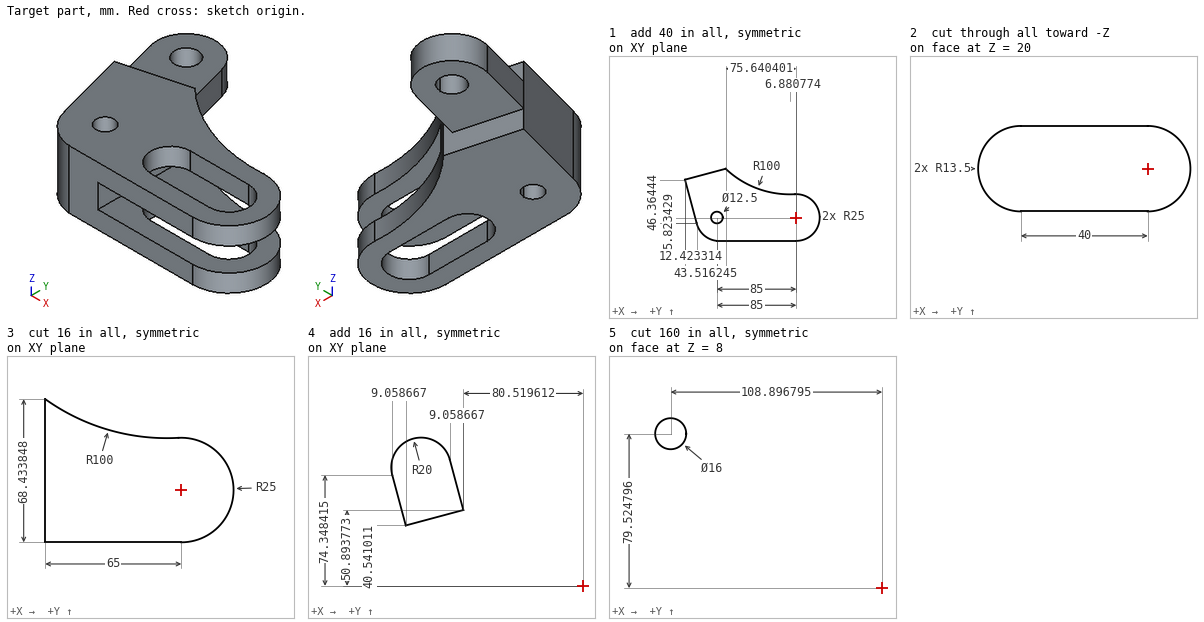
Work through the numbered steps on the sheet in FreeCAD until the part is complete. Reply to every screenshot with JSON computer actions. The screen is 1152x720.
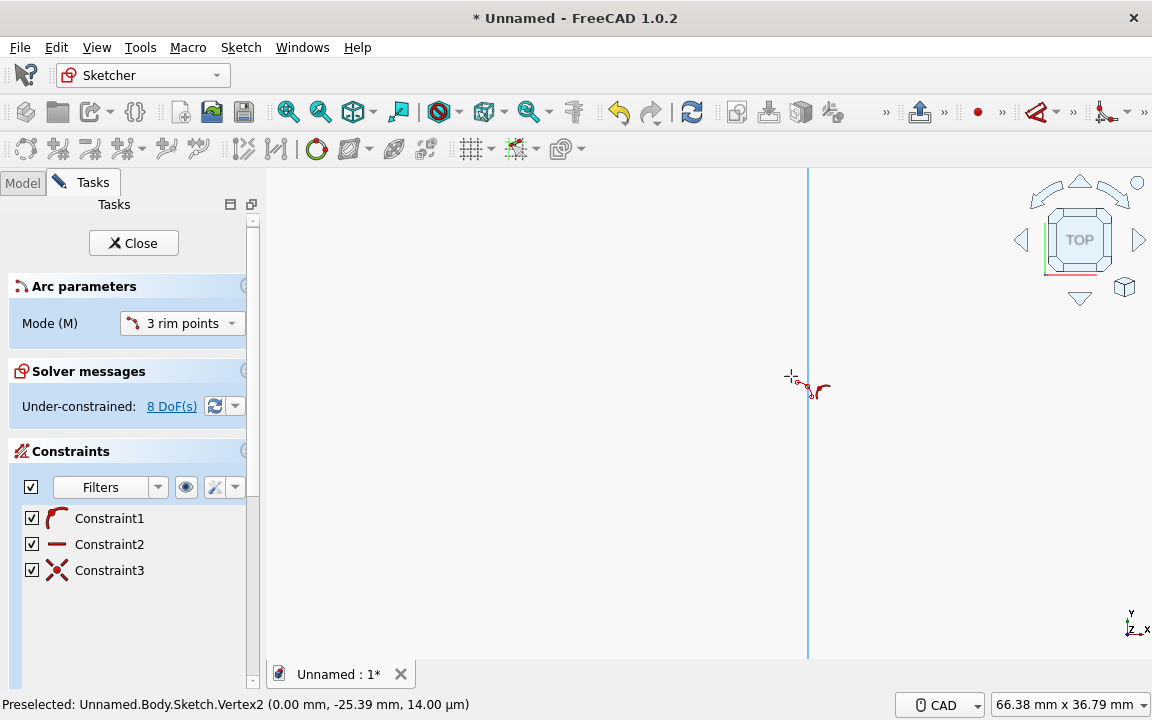
{"action": "left_click", "coordinate": [790, 376]}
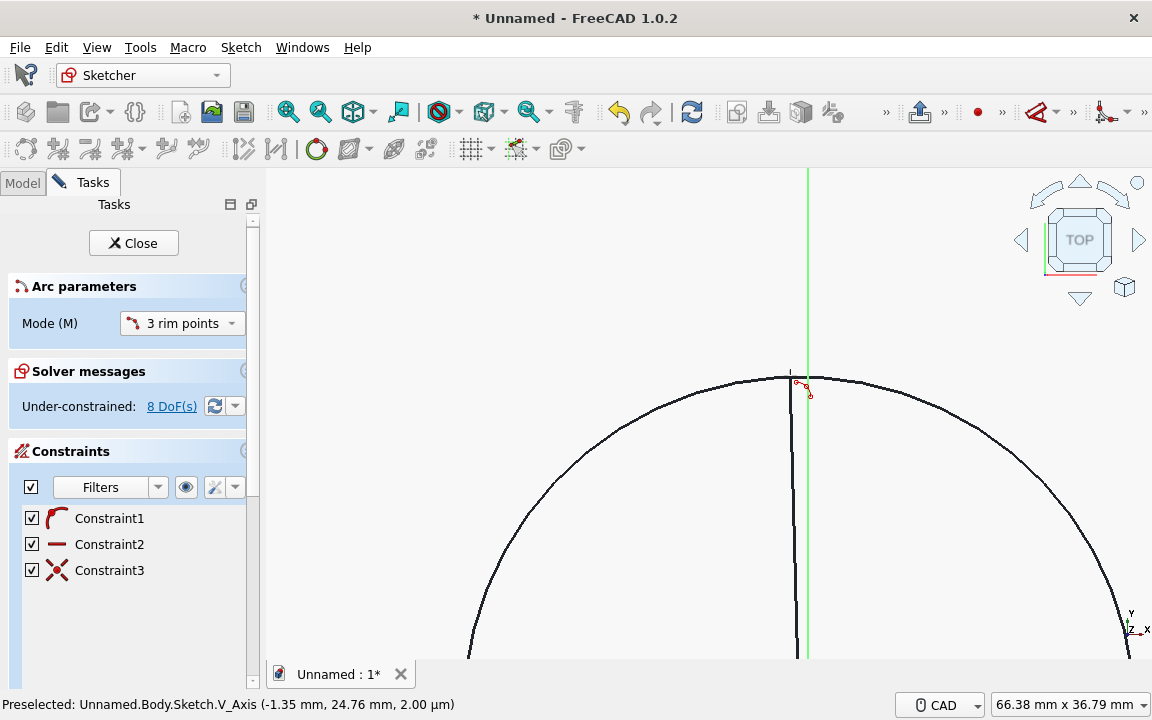
{"action": "scroll", "coordinate": [791, 376], "scroll_direction": "down", "scroll_amount": 7}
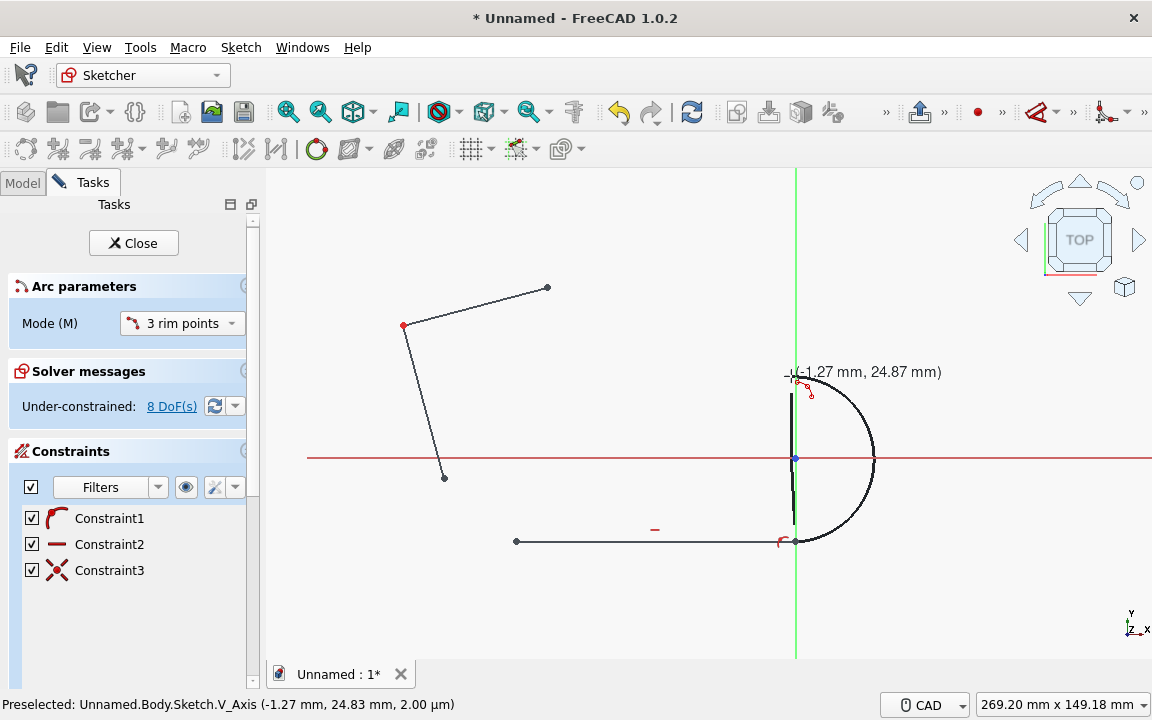
{"action": "left_click", "coordinate": [874, 482]}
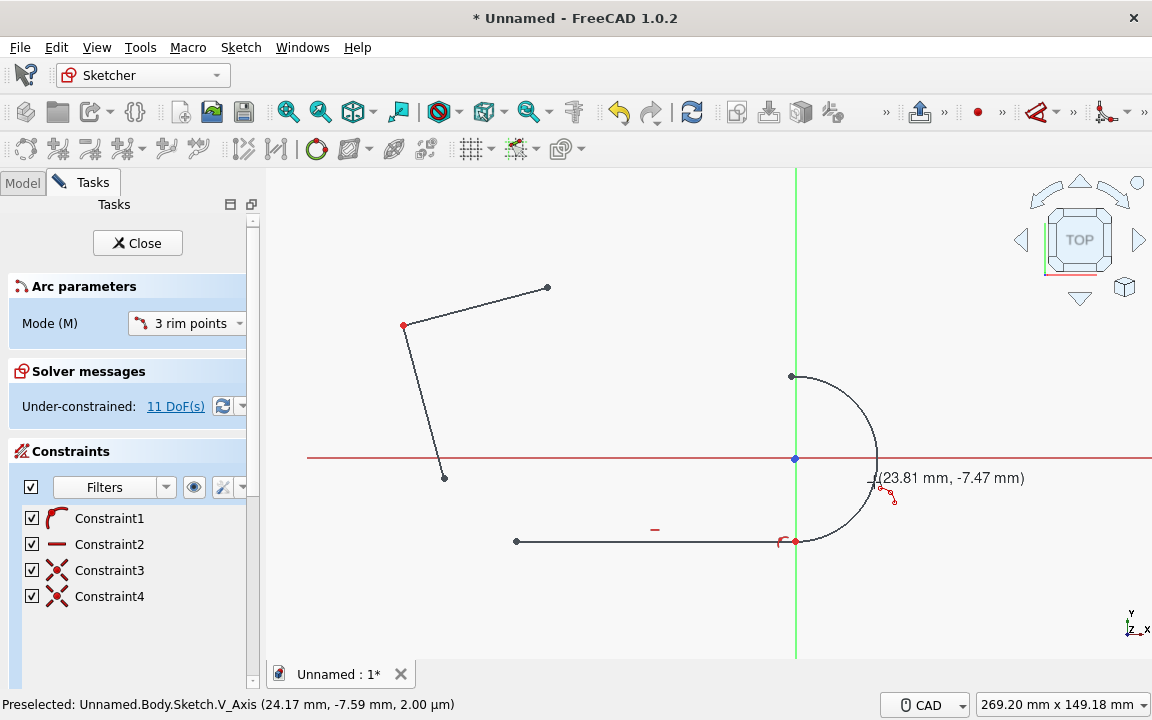
{"action": "scroll", "coordinate": [791, 376], "scroll_direction": "up", "scroll_amount": 7}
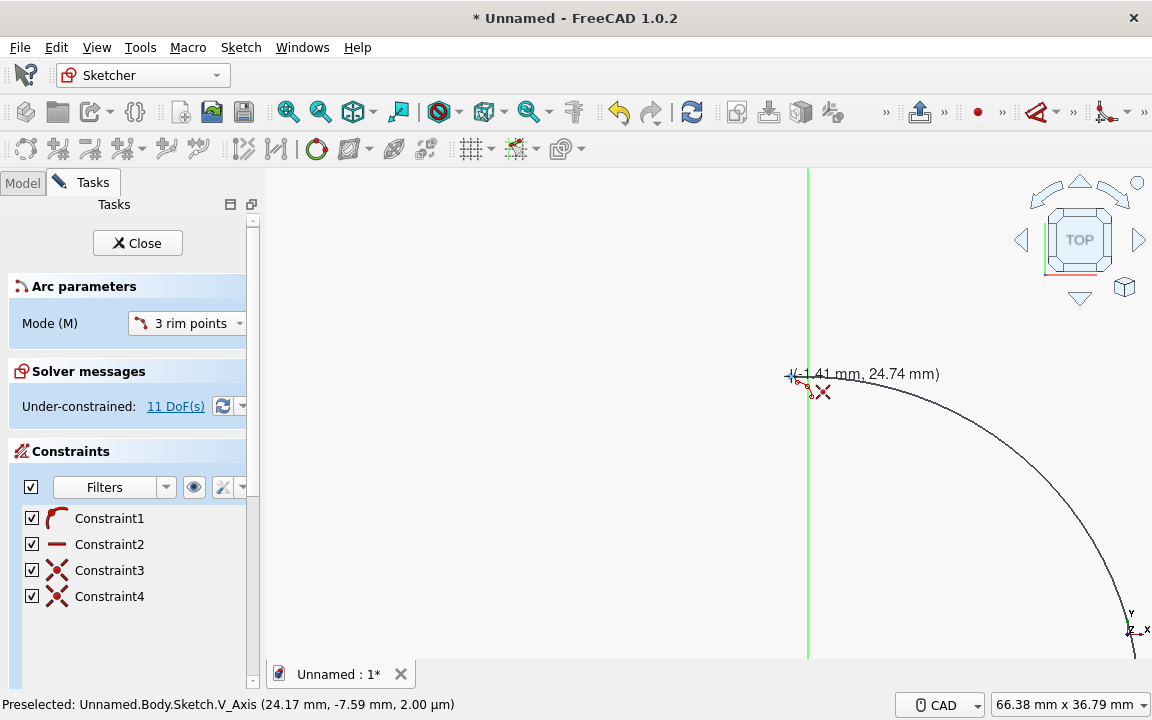
{"action": "left_click", "coordinate": [790, 377]}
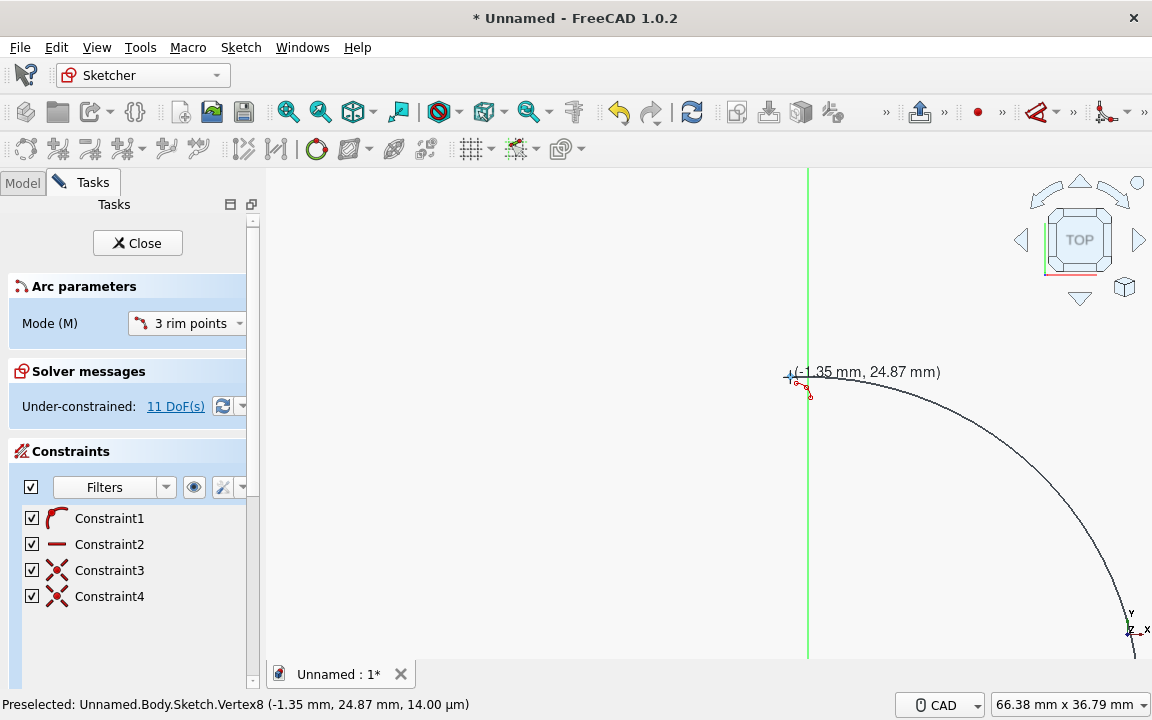
{"action": "scroll", "coordinate": [791, 376], "scroll_direction": "down", "scroll_amount": 7}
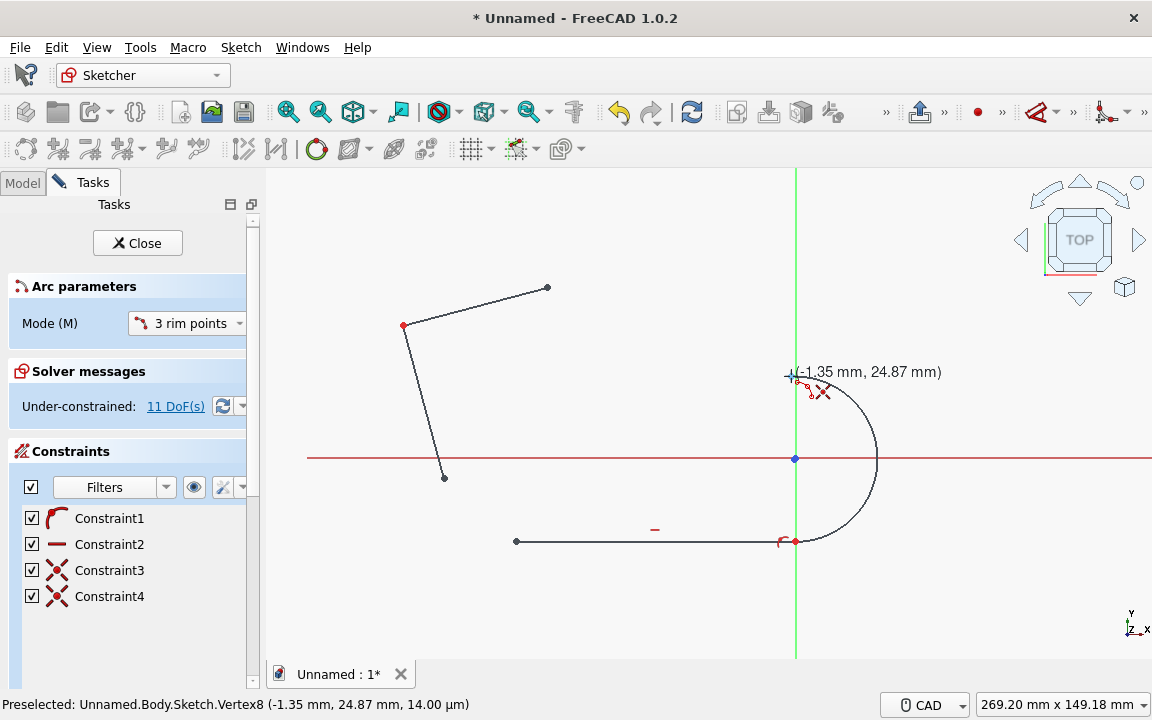
{"action": "left_click", "coordinate": [547, 288]}
{"action": "left_click", "coordinate": [660, 357]}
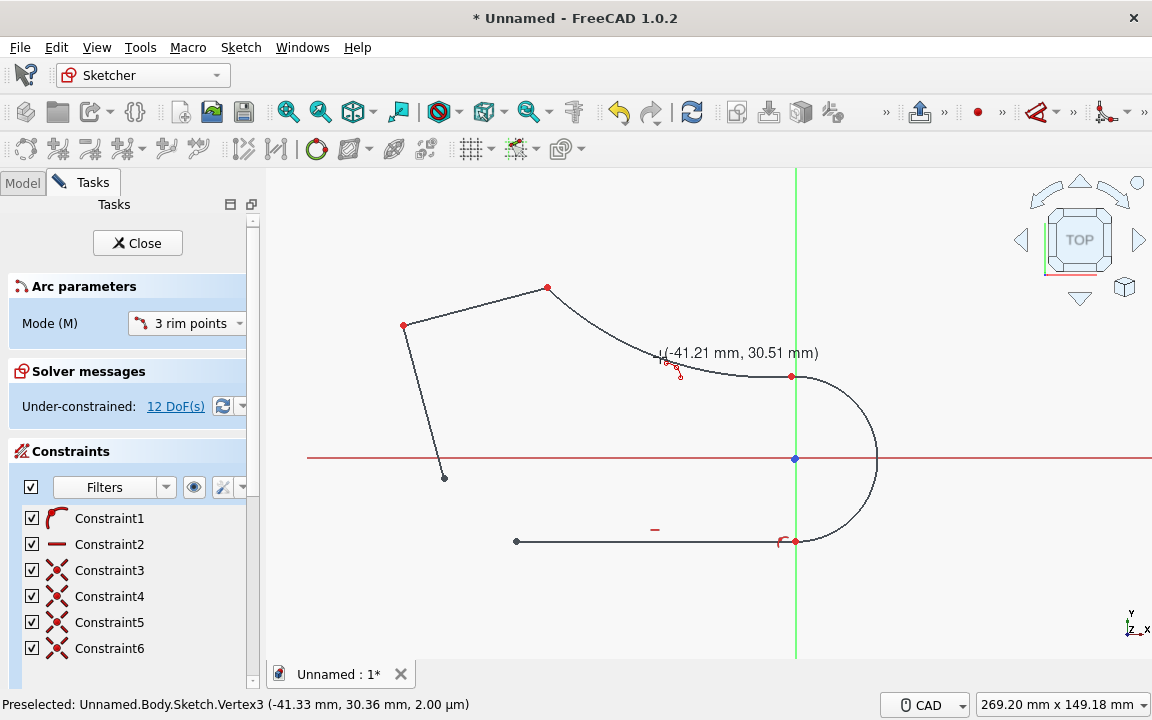
{"action": "left_click", "coordinate": [444, 479]}
{"action": "left_click", "coordinate": [516, 542]}
{"action": "left_click", "coordinate": [470, 521]}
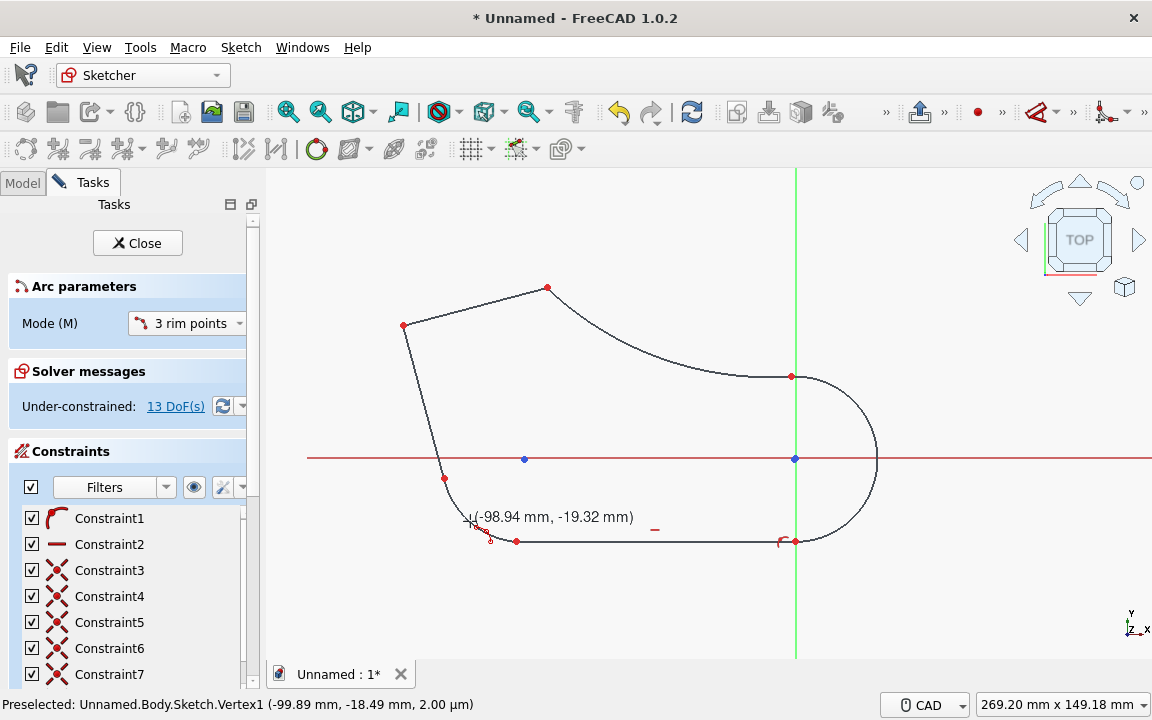
{"action": "key", "text": "g c"}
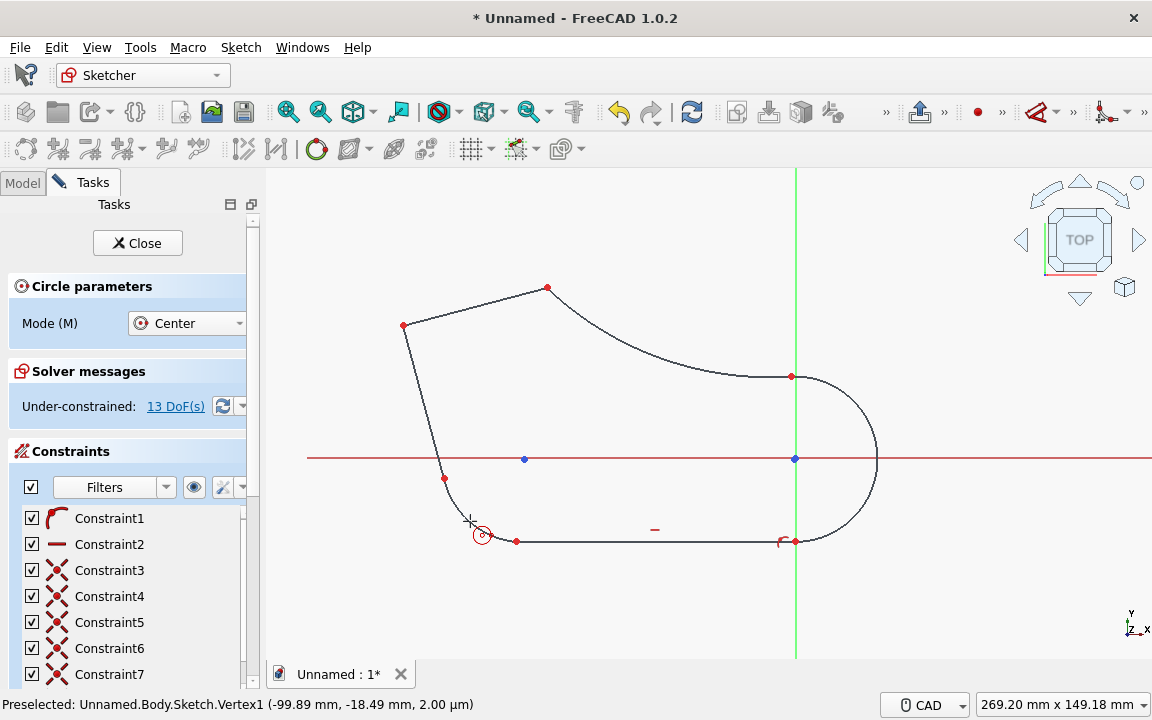
{"action": "scroll", "coordinate": [516, 458], "scroll_direction": "up", "scroll_amount": 4}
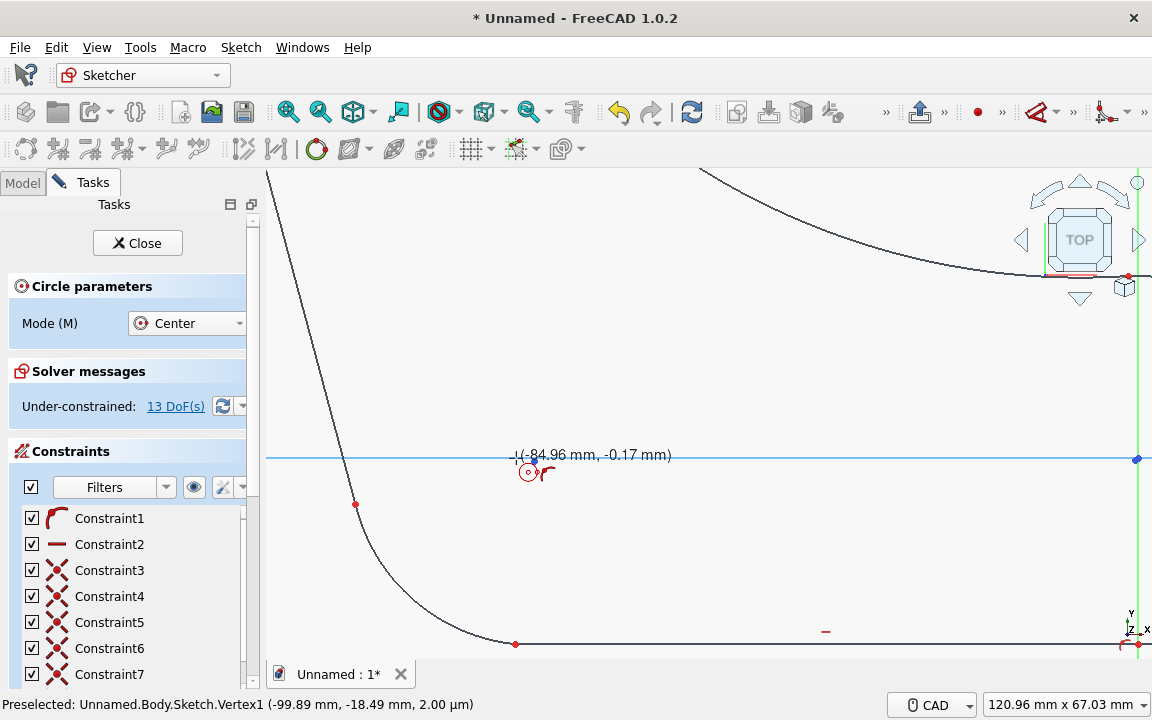
{"action": "left_click", "coordinate": [515, 458]}
{"action": "mouse_move", "coordinate": [548, 426]}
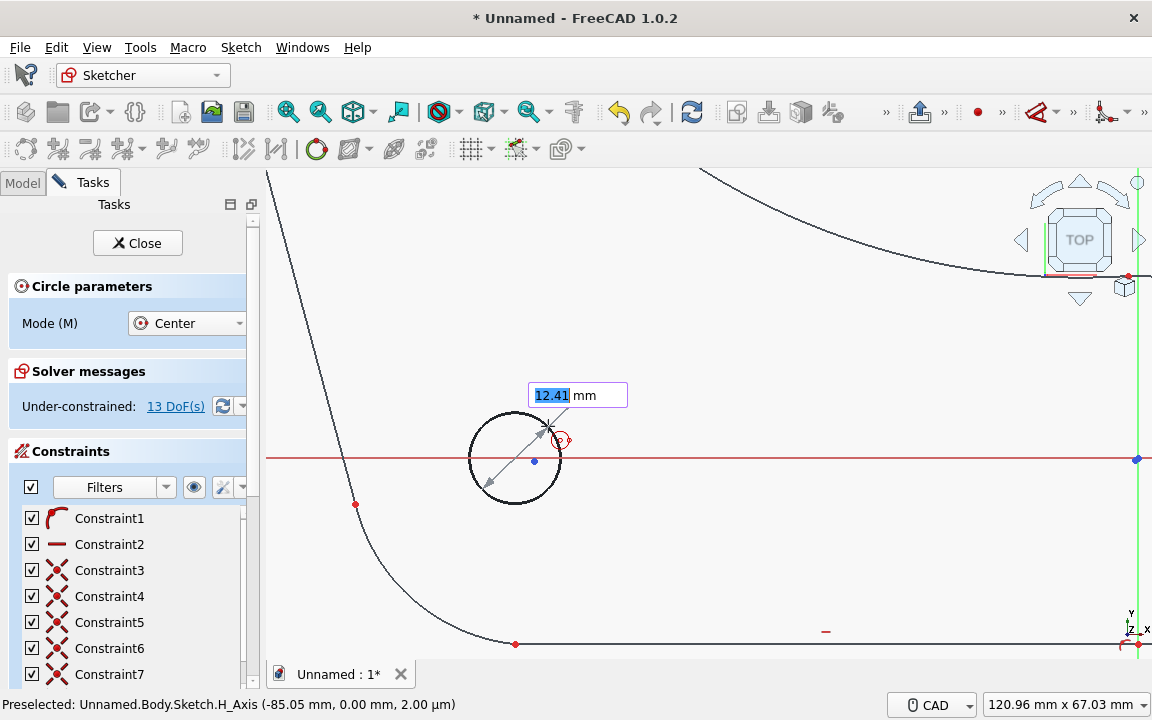
{"action": "type", "text": "12.5"}
{"action": "key", "text": "Return"}
{"action": "key", "text": "Escape"}